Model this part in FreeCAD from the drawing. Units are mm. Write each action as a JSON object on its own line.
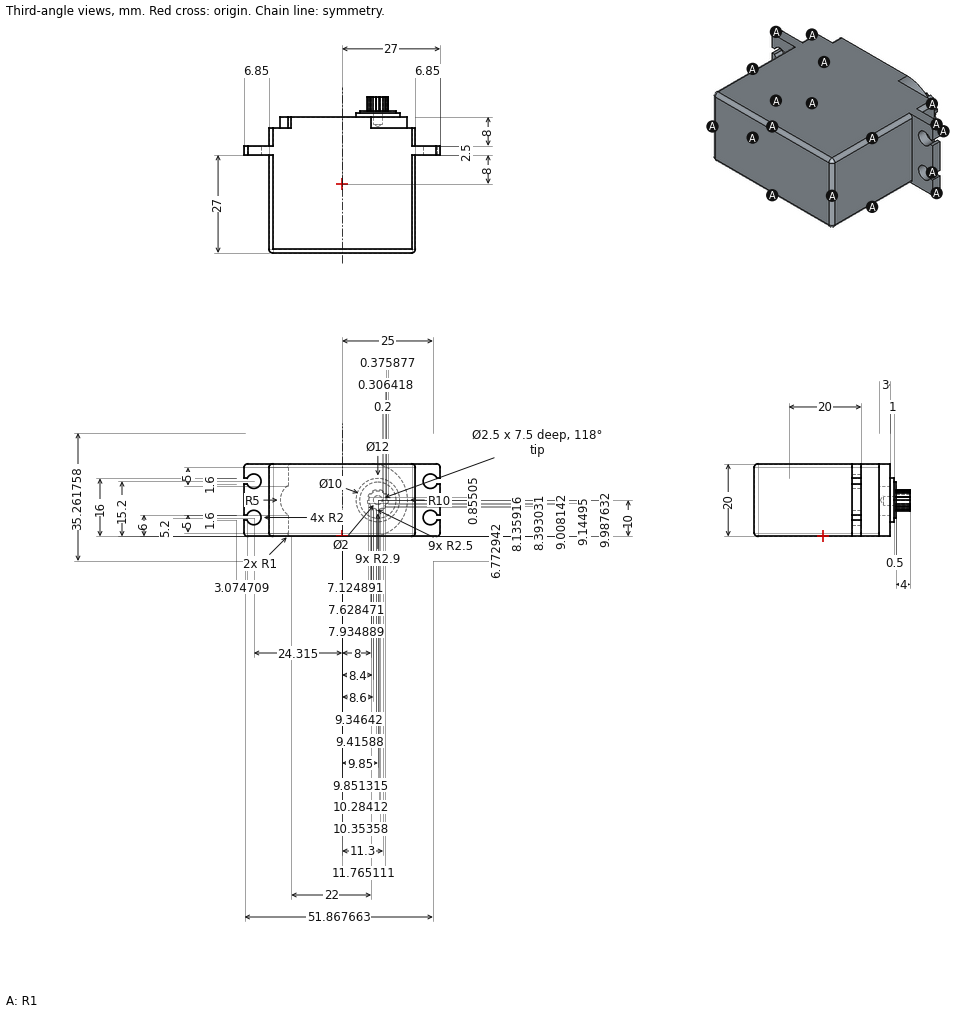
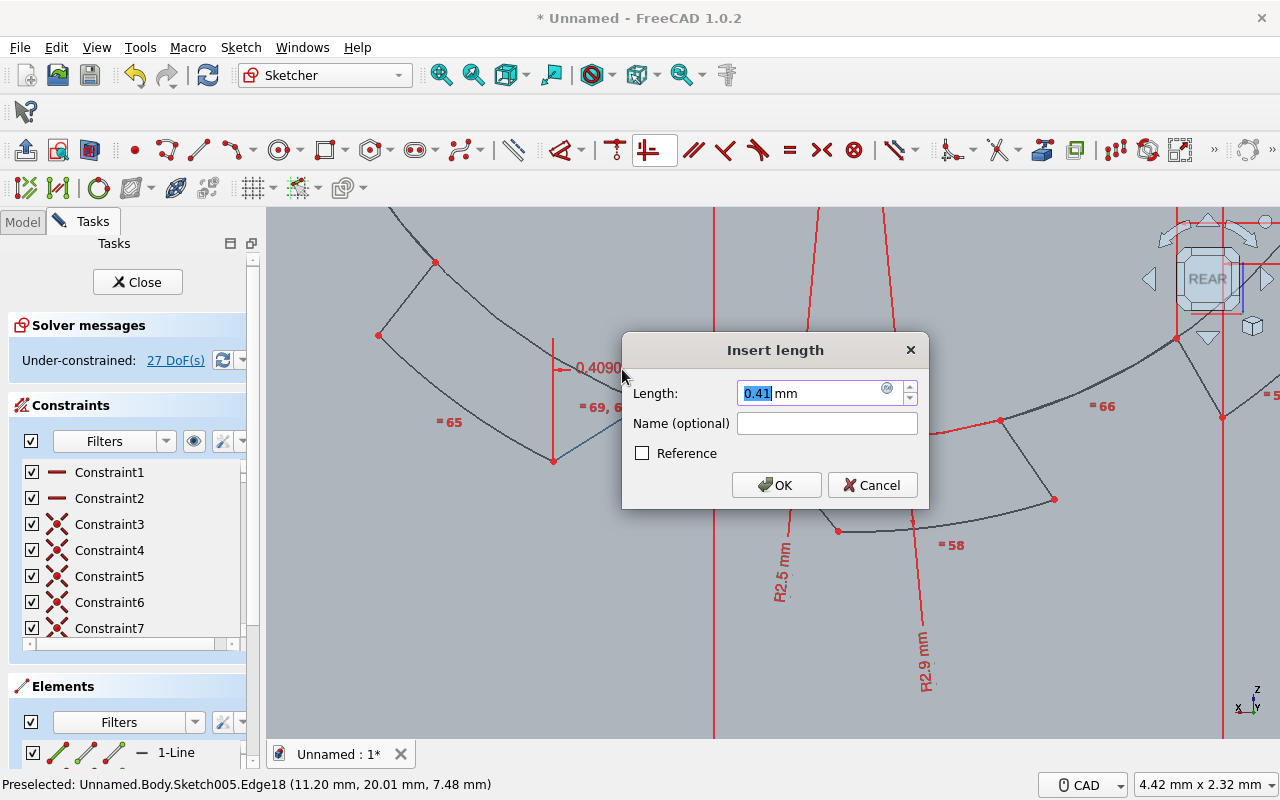
{"action": "type", "text": "0.2"}
{"action": "key", "text": "Return"}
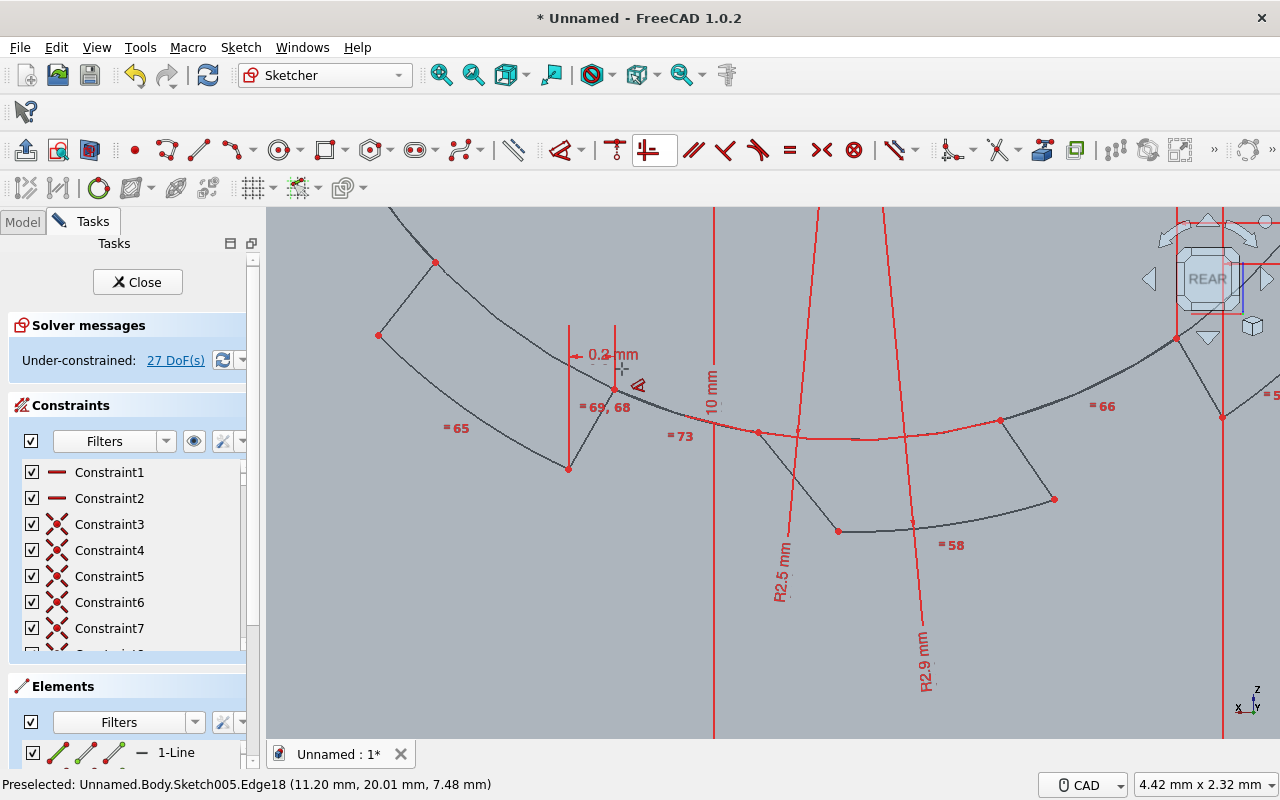
{"action": "scroll", "coordinate": [582, 446], "scroll_direction": "down", "scroll_amount": 11}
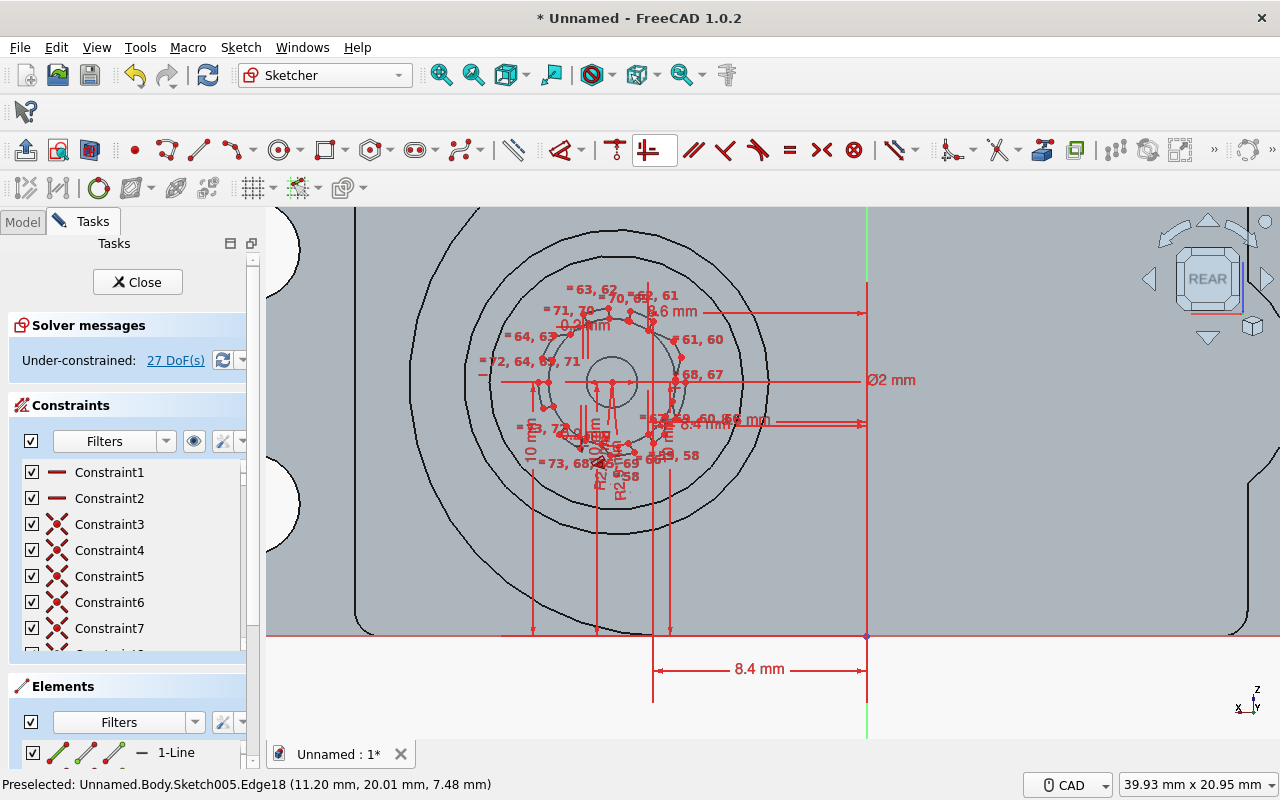
{"action": "left_click", "coordinate": [612, 382]}
{"action": "left_click", "coordinate": [681, 670]}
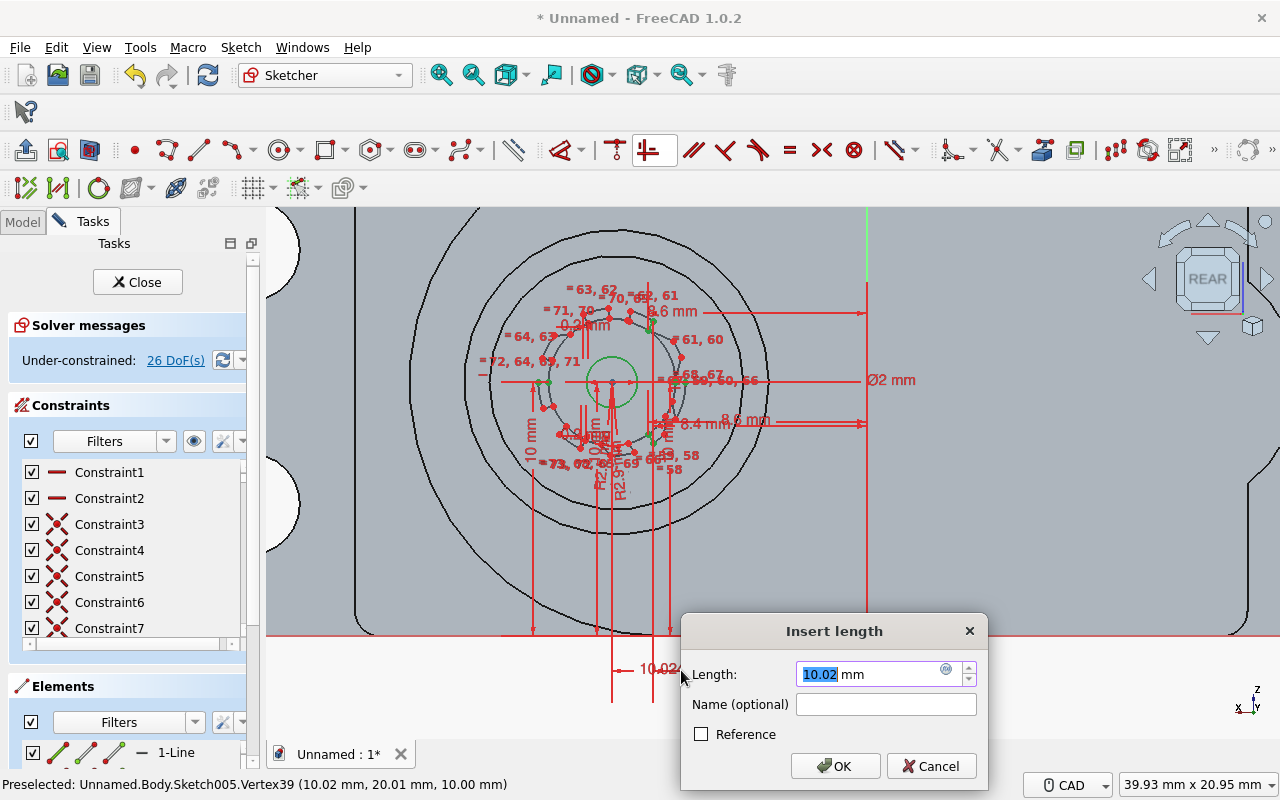
{"action": "type", "text": "9.85"}
{"action": "key", "text": "Return"}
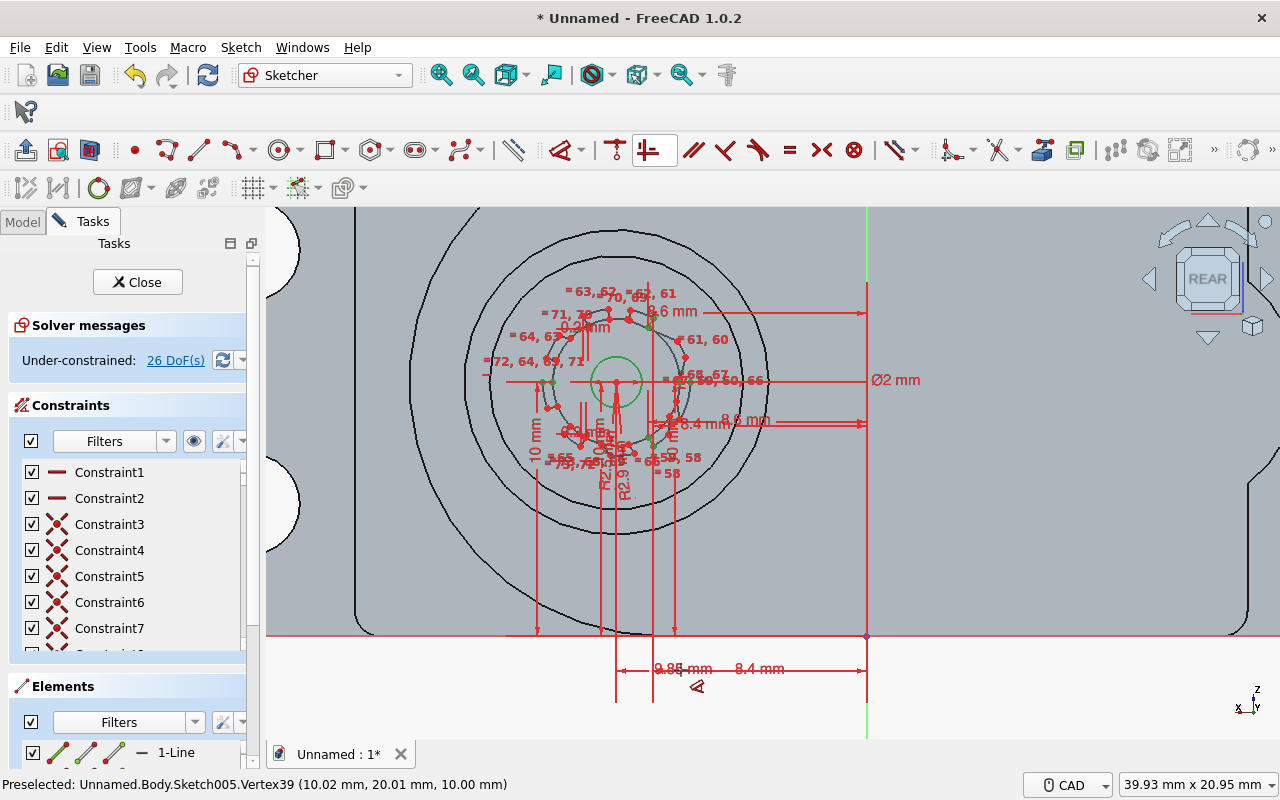
{"action": "left_click", "coordinate": [583, 317]}
{"action": "left_click", "coordinate": [725, 283]}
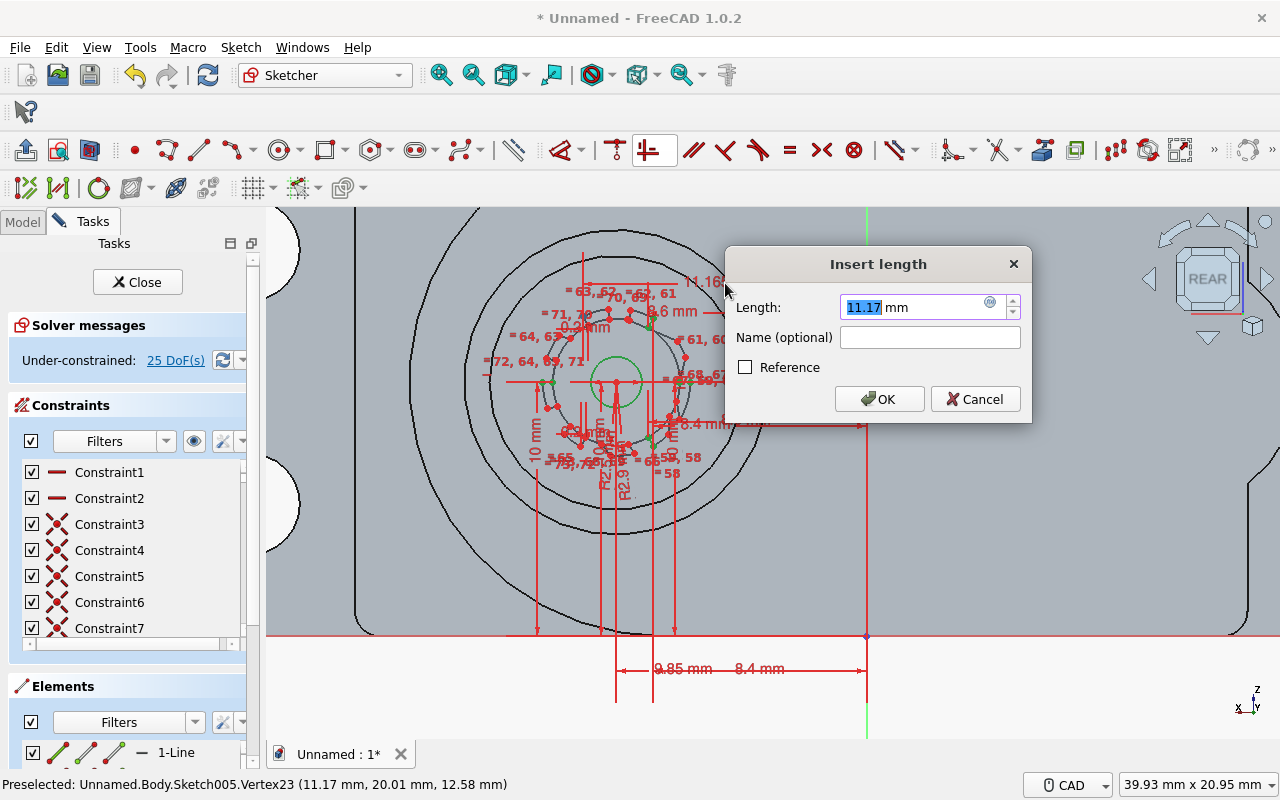
{"action": "type", "text": "11.3"}
{"action": "key", "text": "Return"}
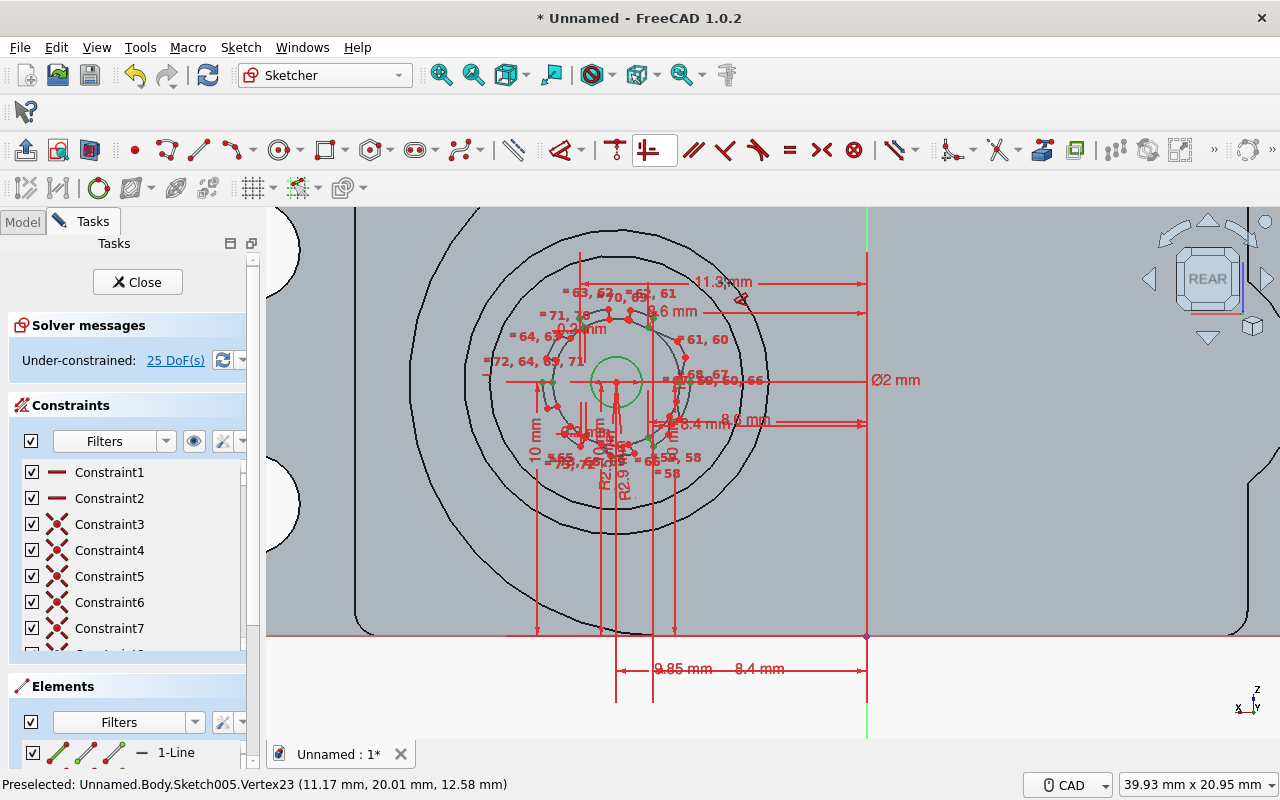
{"action": "left_click", "coordinate": [581, 447]}
{"action": "left_click", "coordinate": [824, 413]}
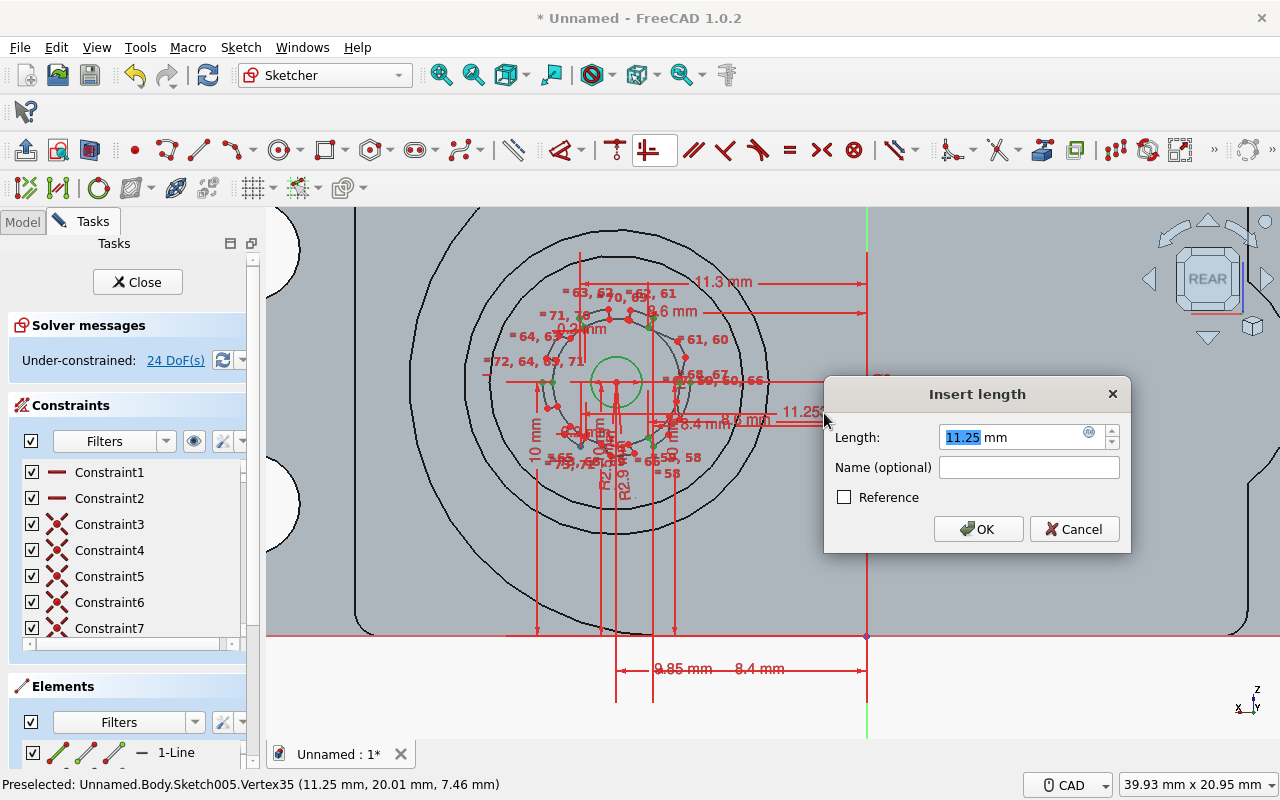
{"action": "type", "text": "11.3"}
{"action": "key", "text": "Return"}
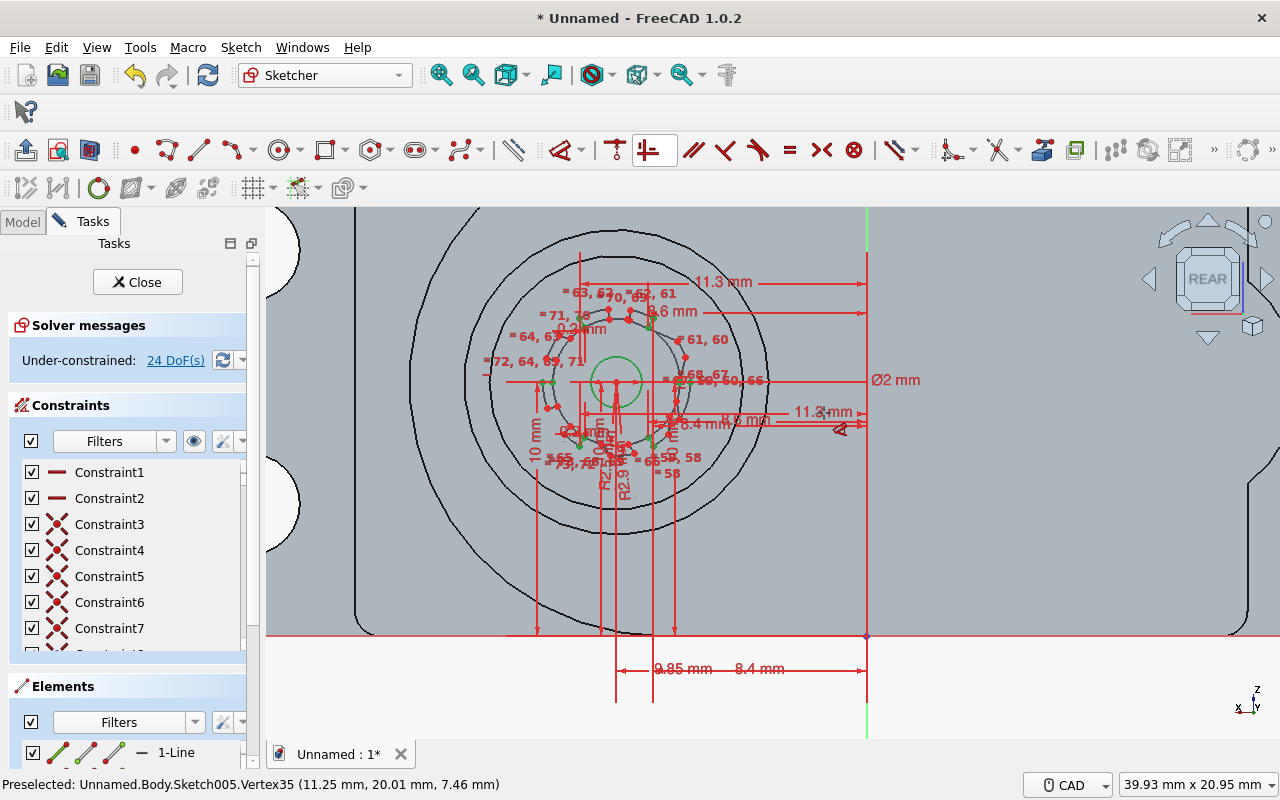
{"action": "left_click", "coordinate": [635, 454]}
{"action": "left_click", "coordinate": [832, 670]}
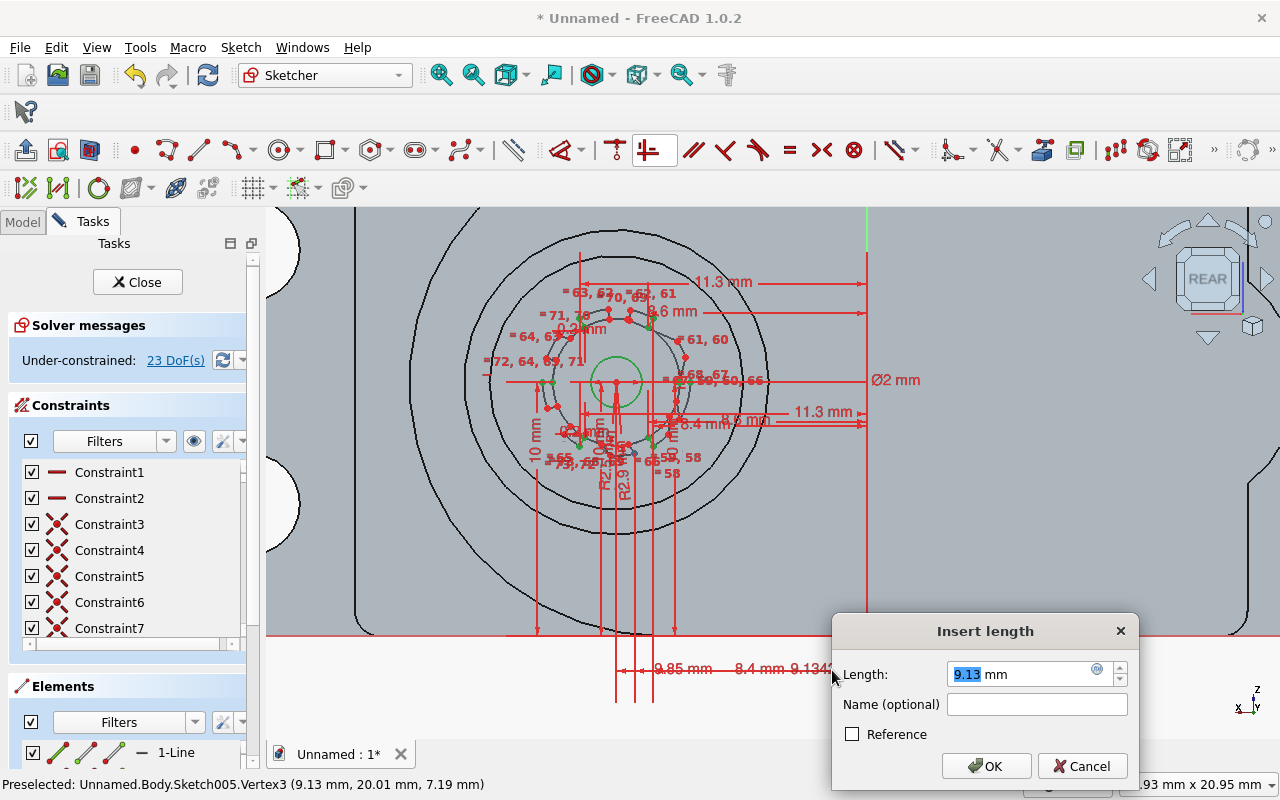
{"action": "type", "text": "9.34642"}
{"action": "key", "text": "Return"}